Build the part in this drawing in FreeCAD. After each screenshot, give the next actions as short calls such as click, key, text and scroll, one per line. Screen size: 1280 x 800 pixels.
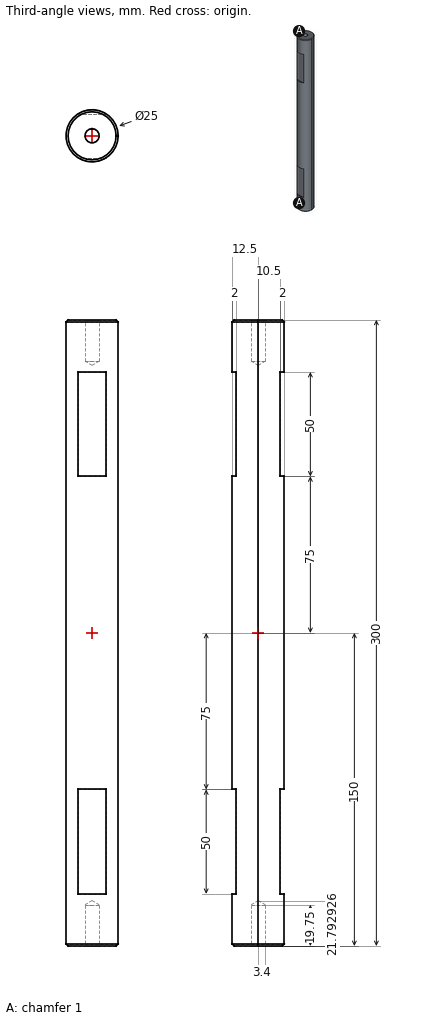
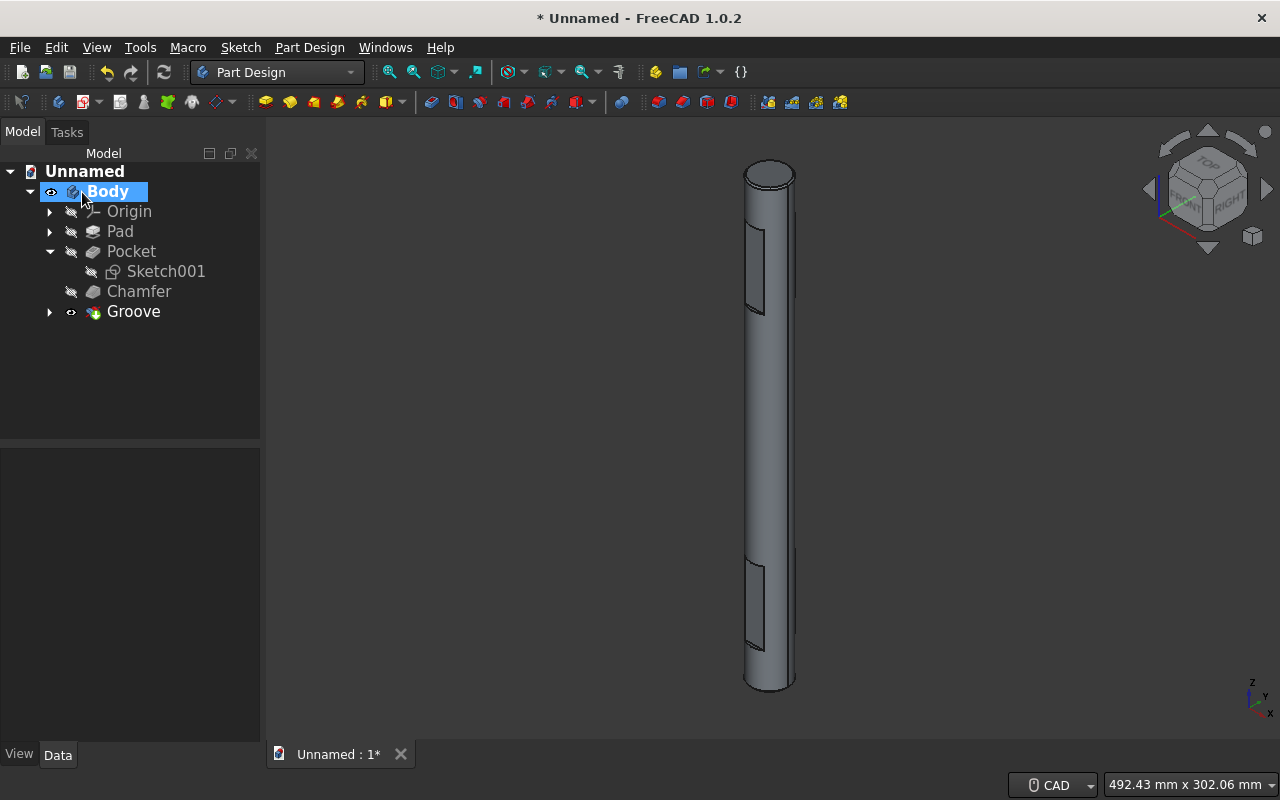
click(116, 312)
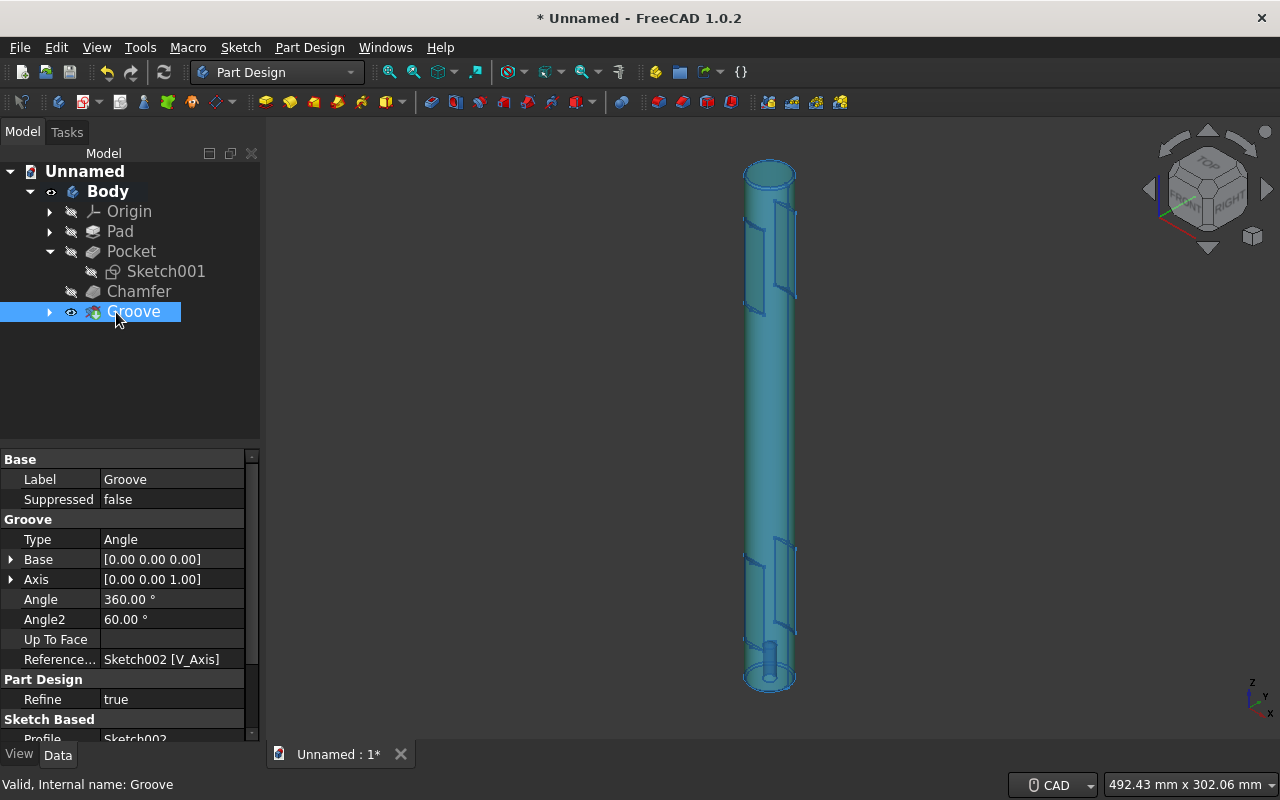
click(768, 102)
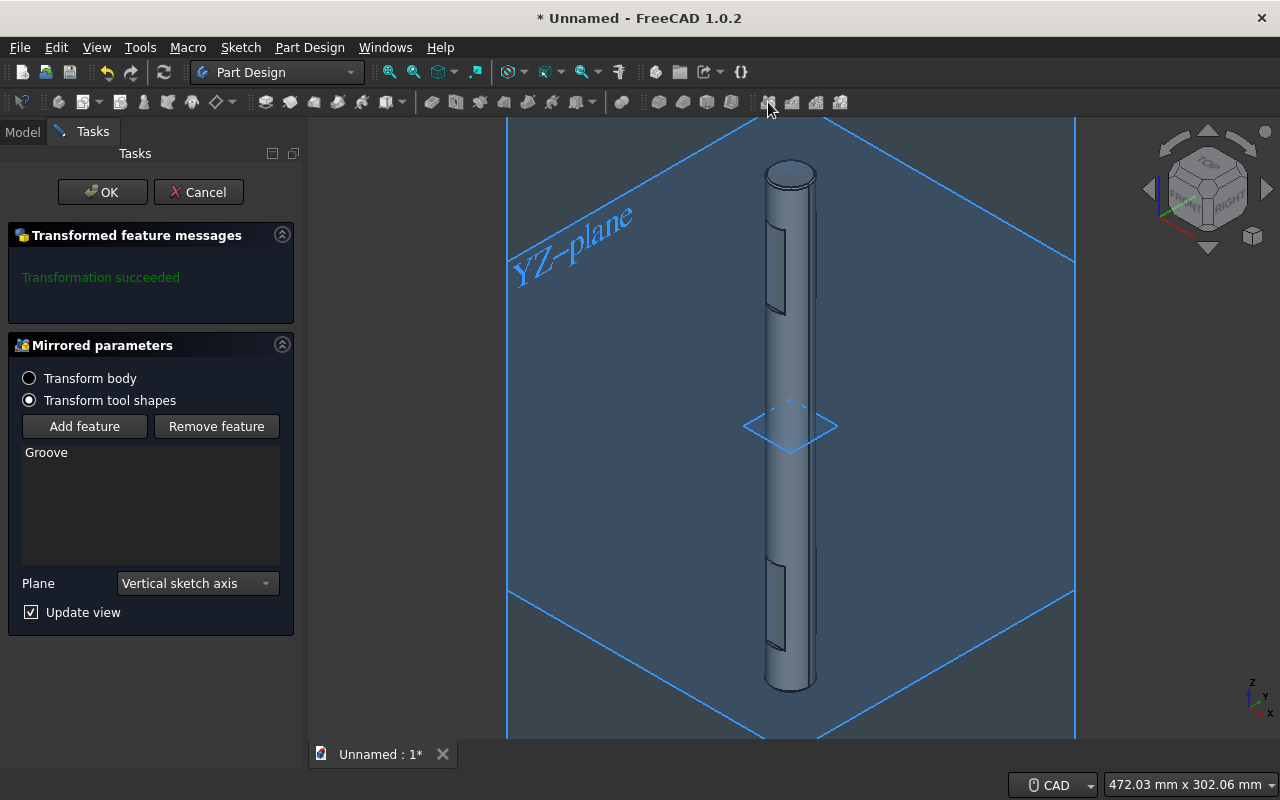
click(198, 584)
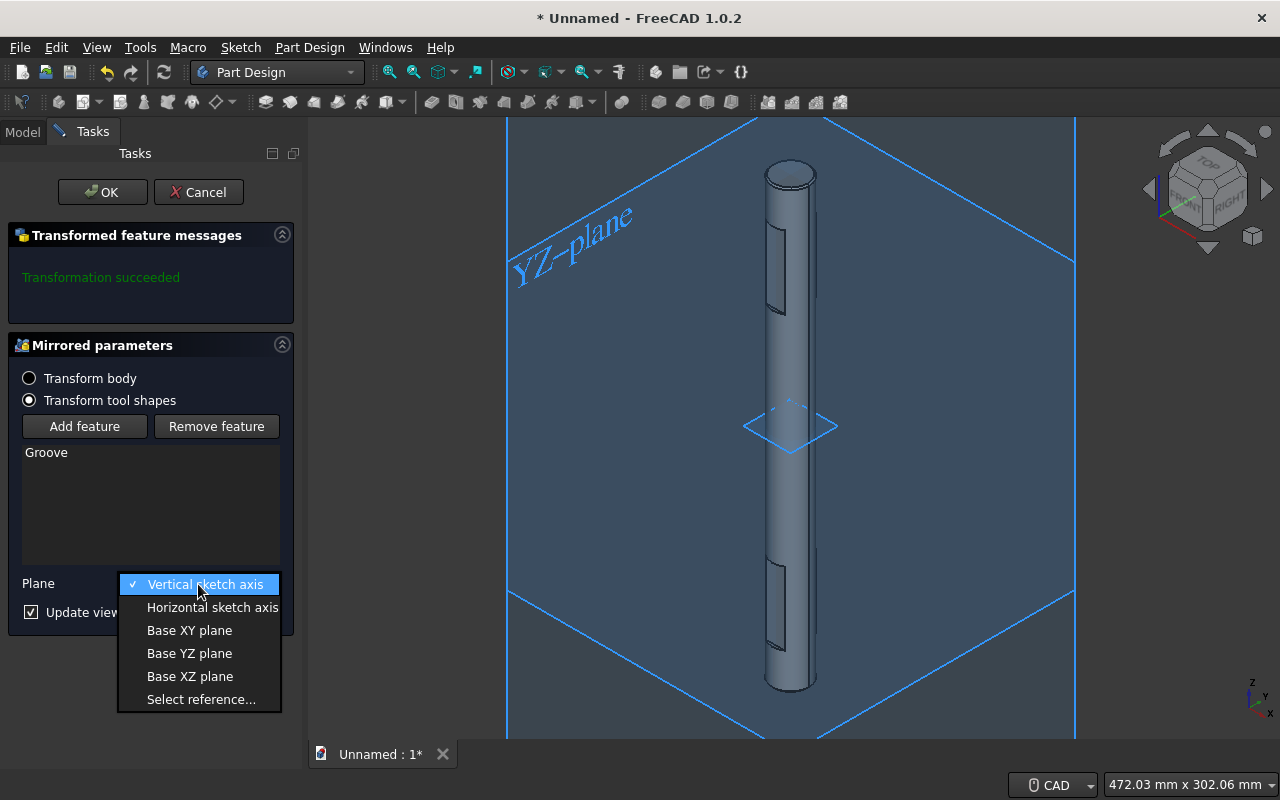
click(198, 630)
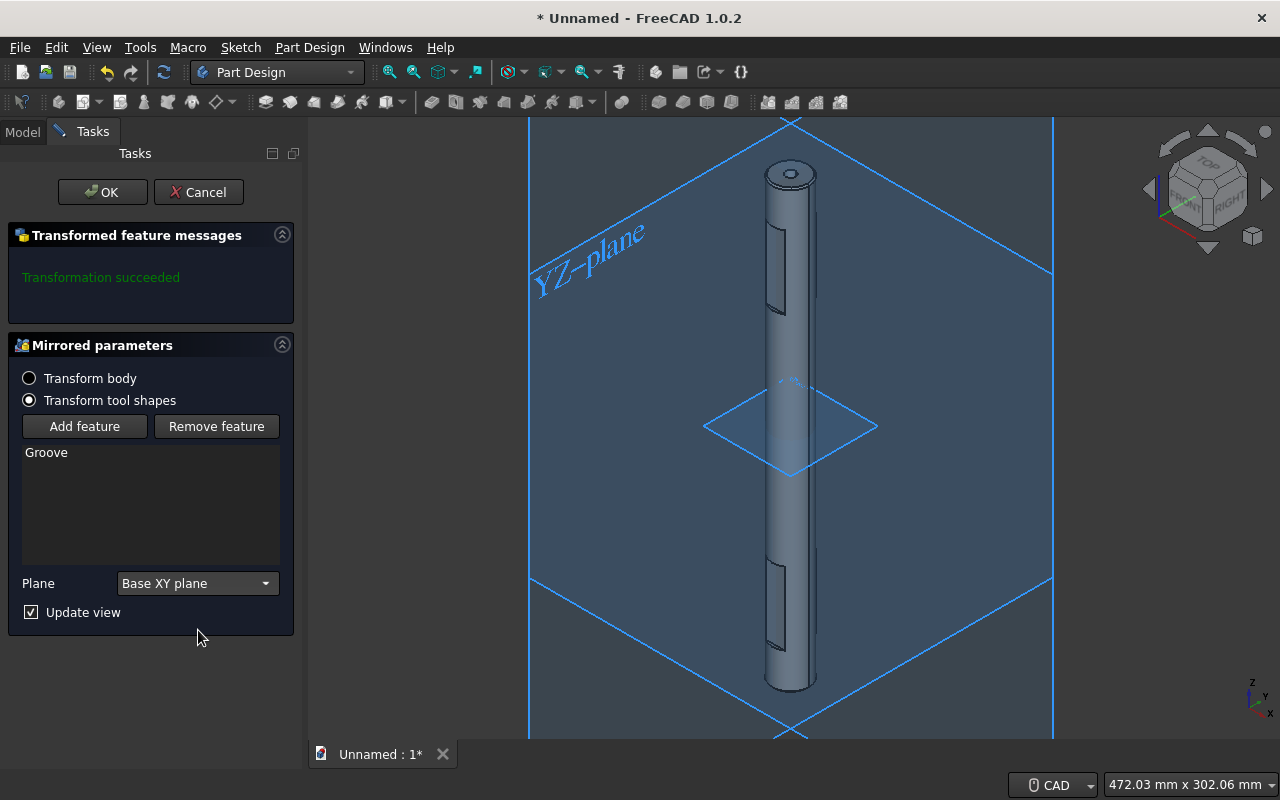
click(103, 192)